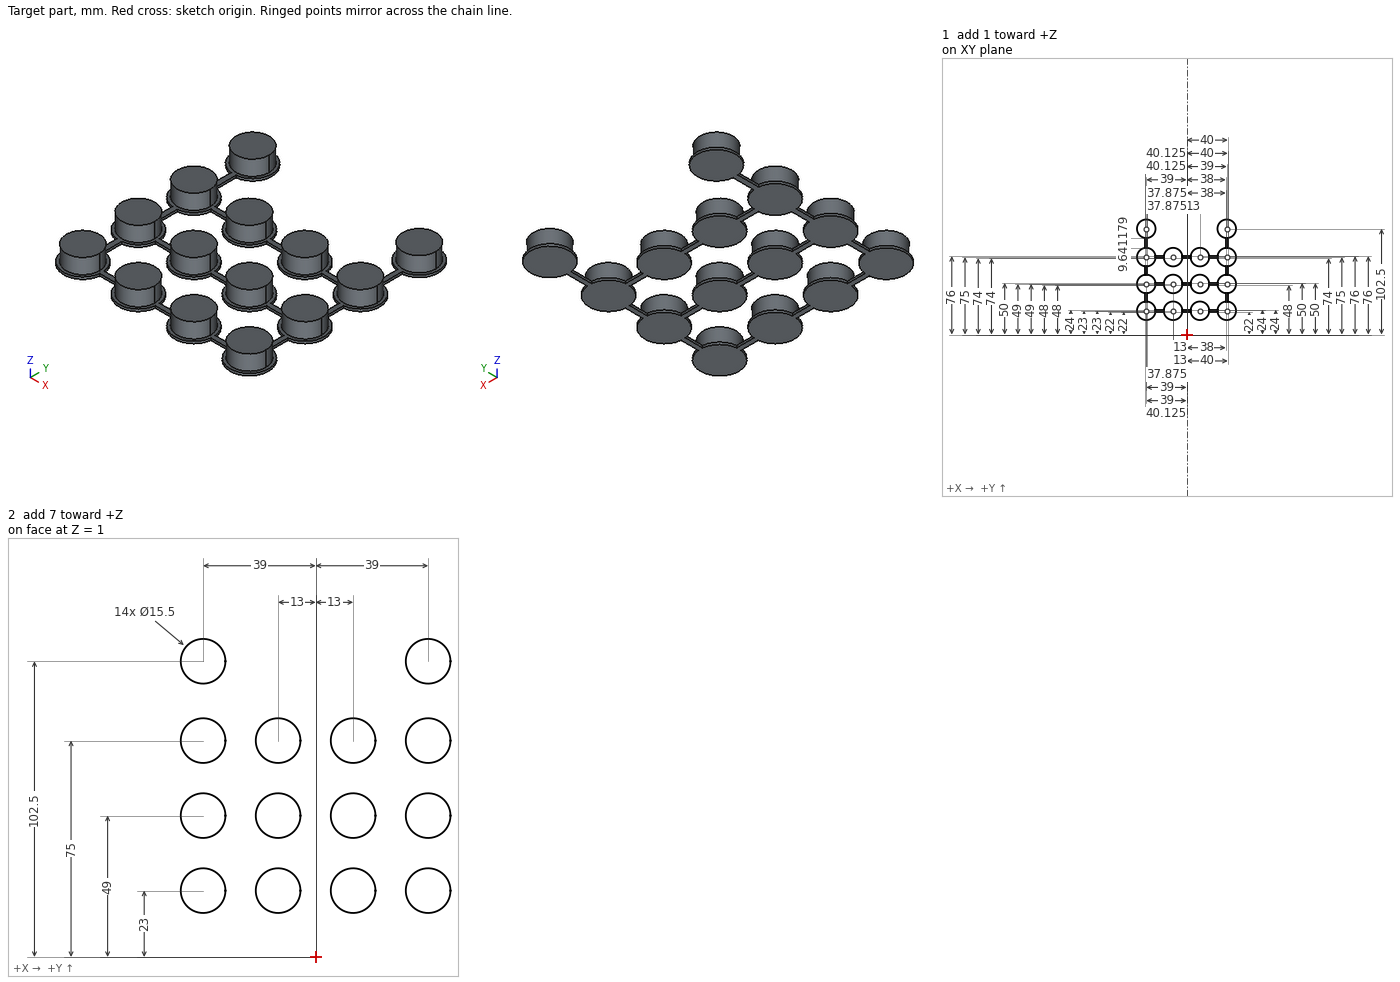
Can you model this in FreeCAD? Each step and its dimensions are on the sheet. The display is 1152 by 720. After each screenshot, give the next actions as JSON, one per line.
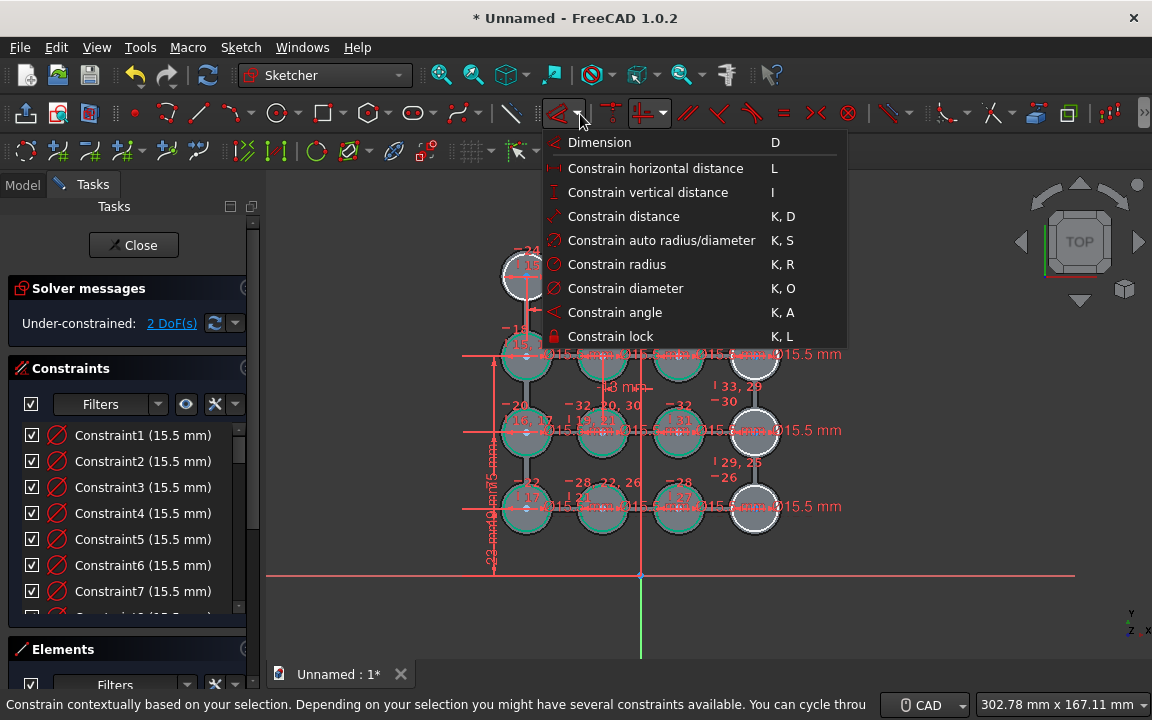
{"action": "left_click", "coordinate": [695, 168]}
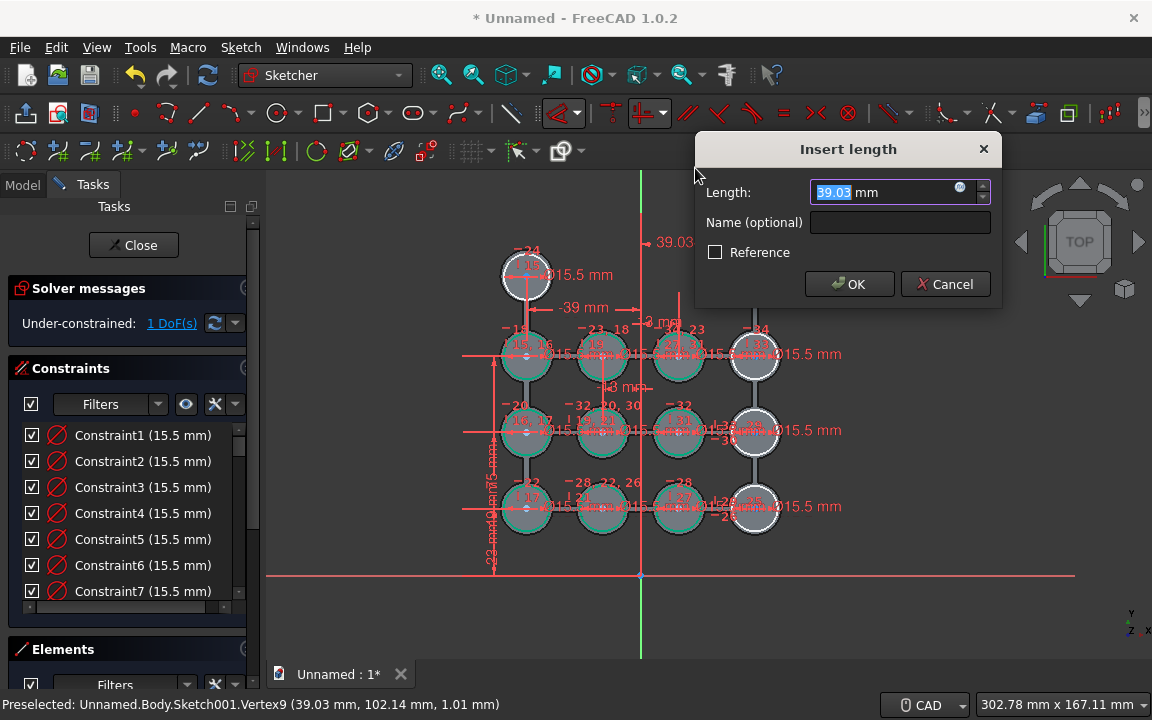
{"action": "type", "text": "39"}
{"action": "key", "text": "Return"}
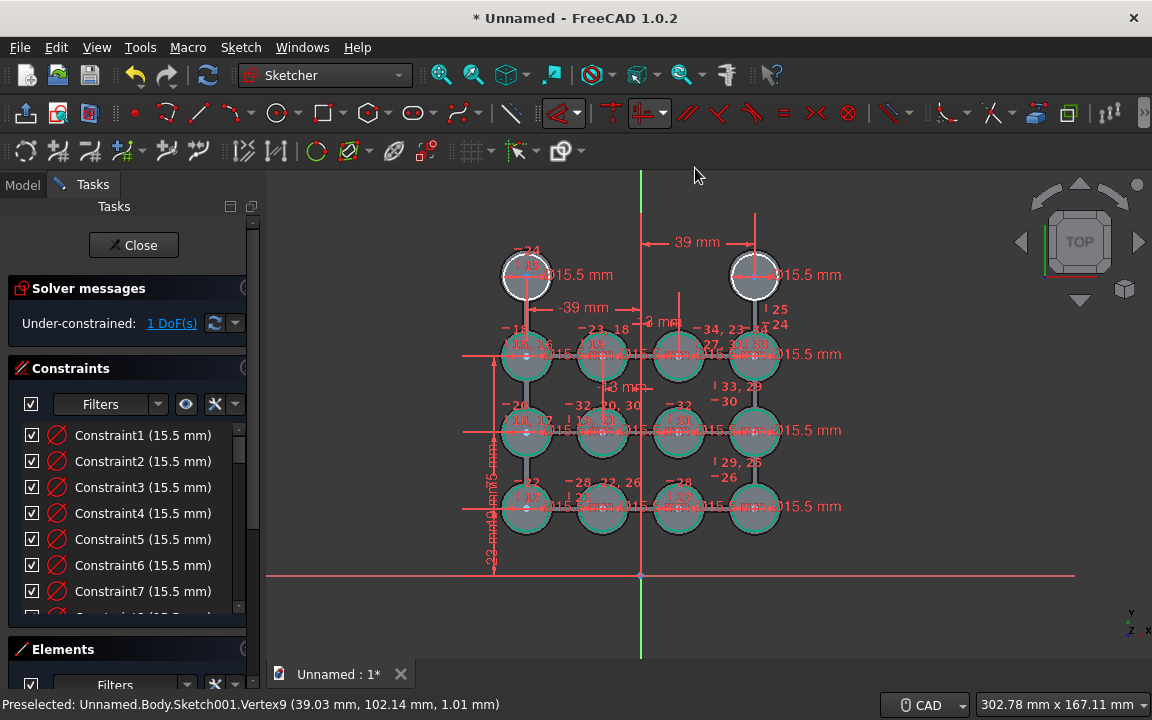
{"action": "left_click", "coordinate": [527, 277]}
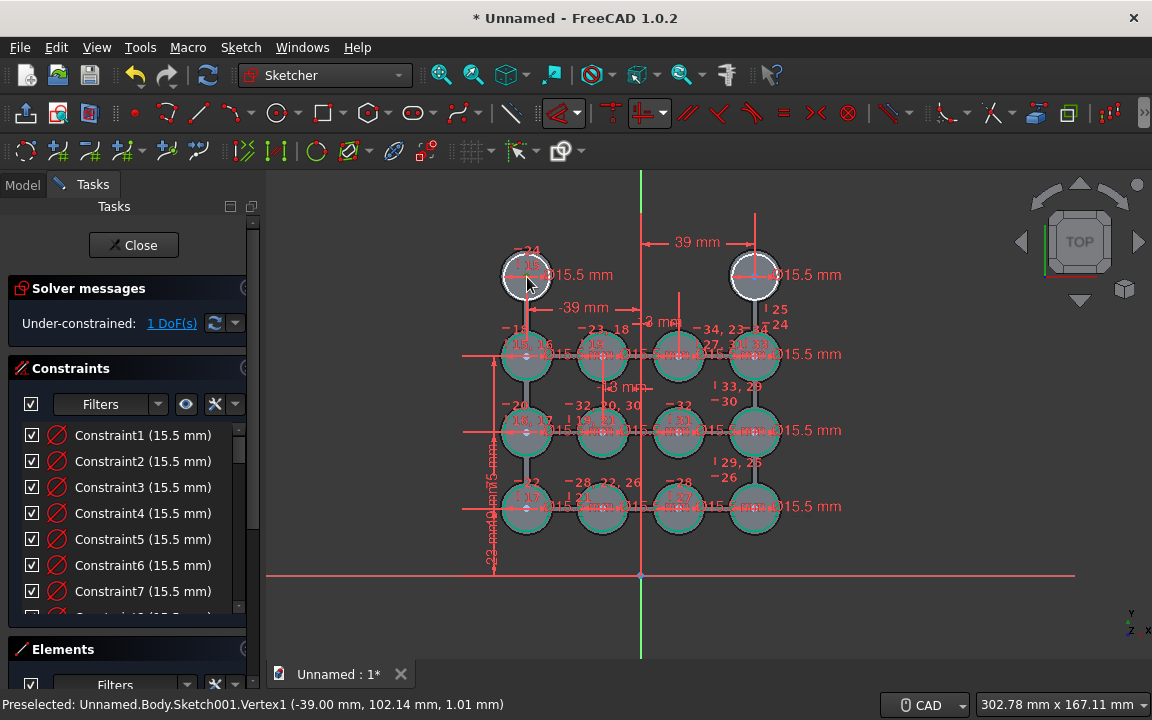
{"action": "left_click", "coordinate": [580, 114]}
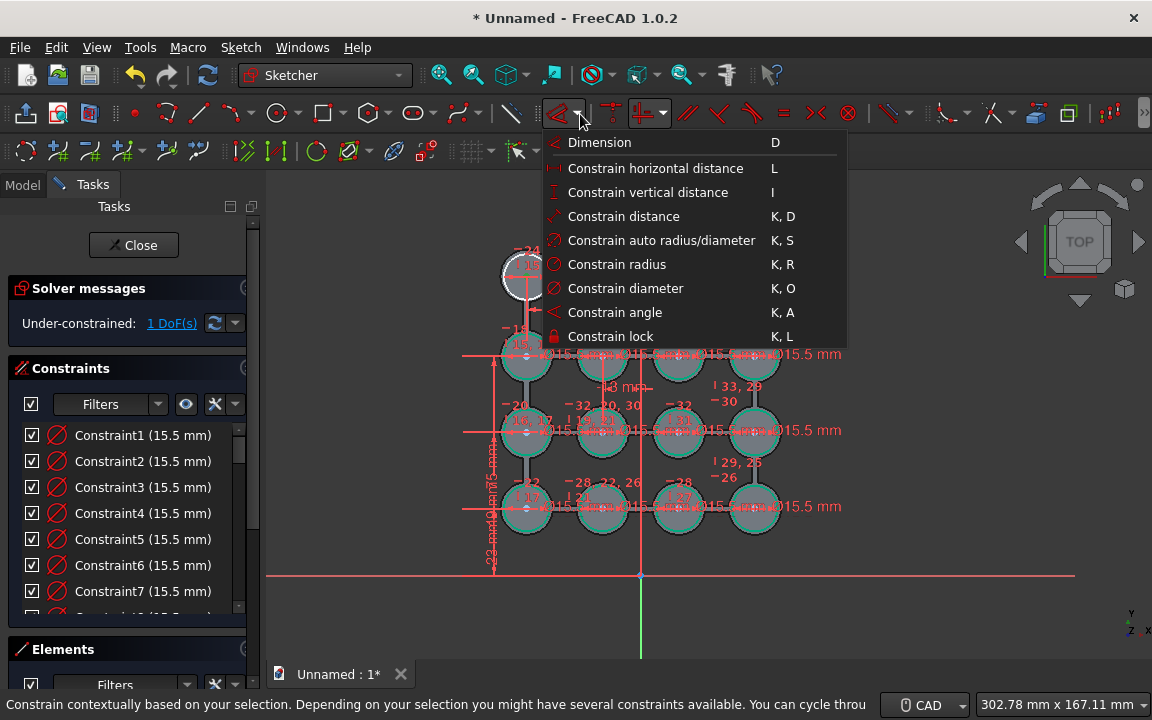
{"action": "left_click", "coordinate": [695, 192]}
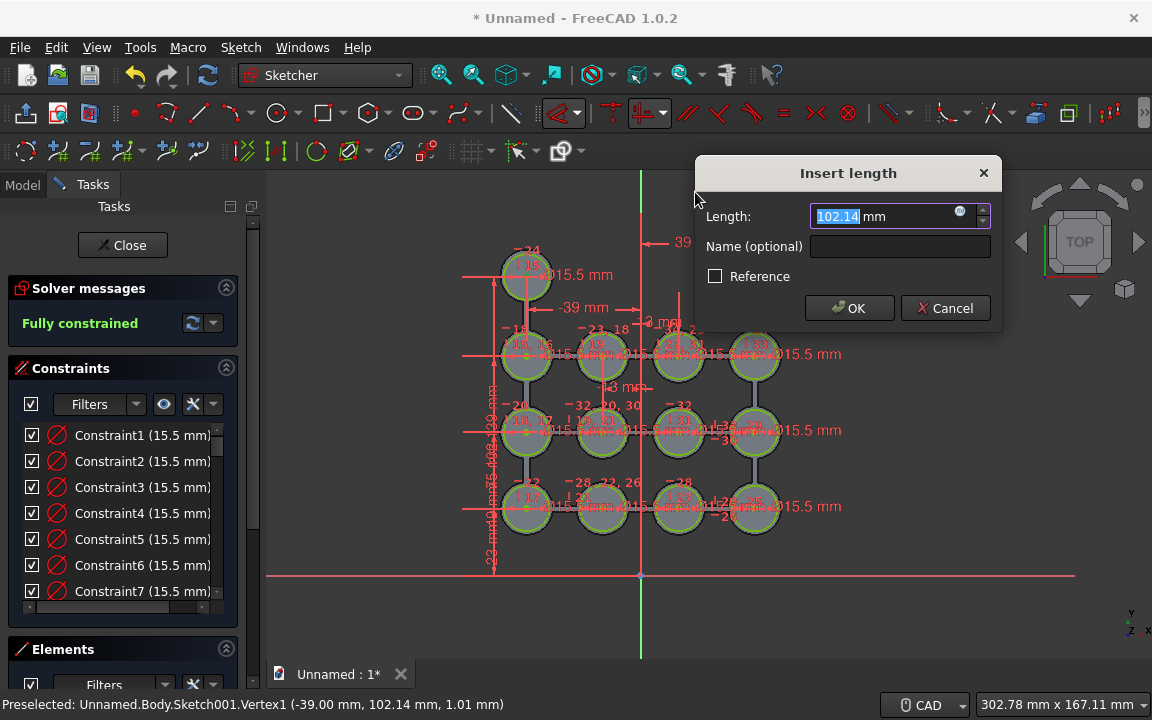
{"action": "type", "text": "102.5"}
{"action": "key", "text": "Return"}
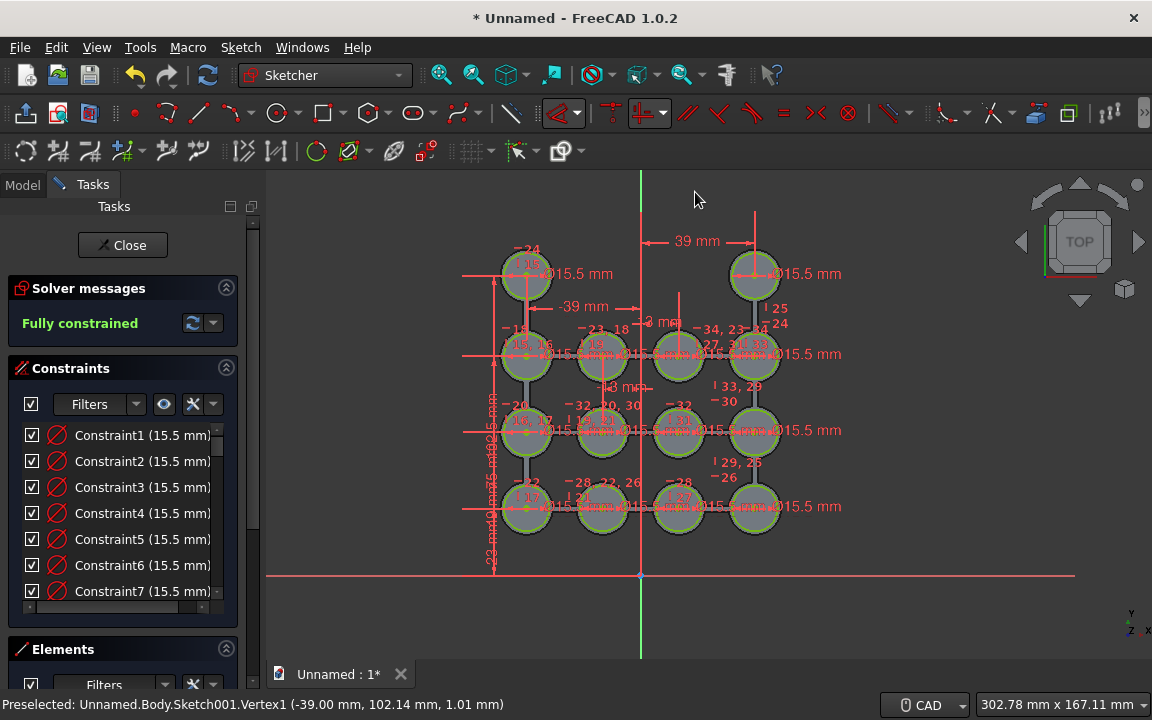
{"action": "left_click", "coordinate": [123, 245]}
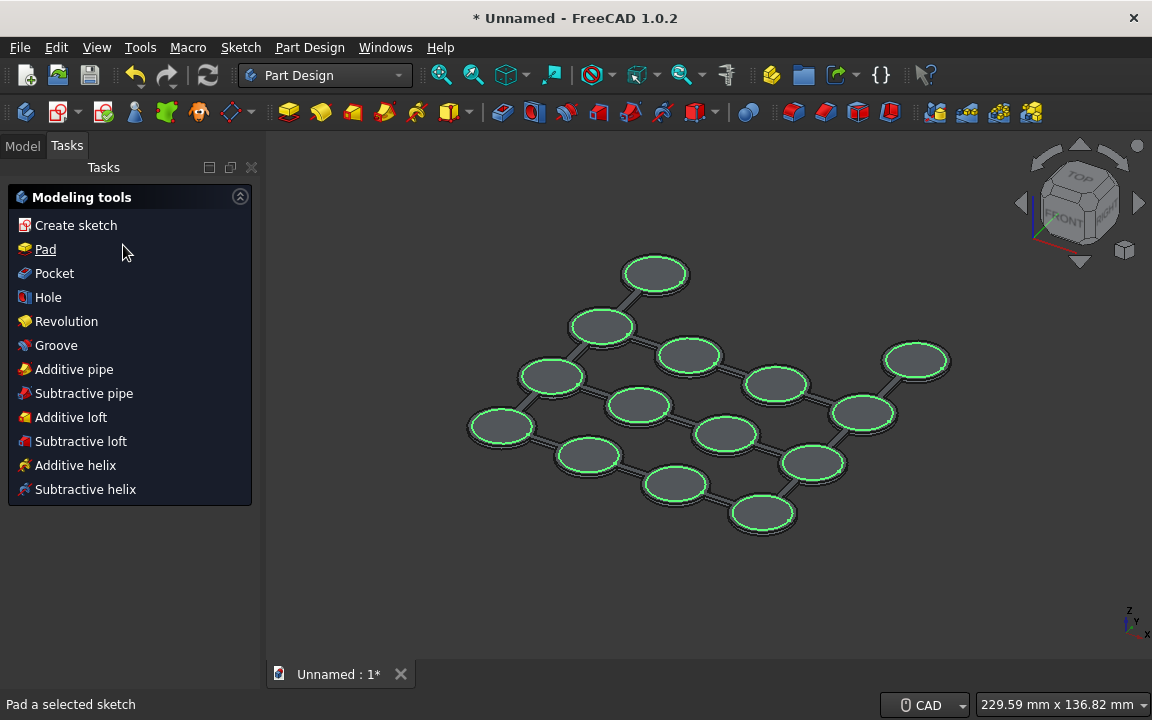
{"action": "left_click", "coordinate": [290, 112]}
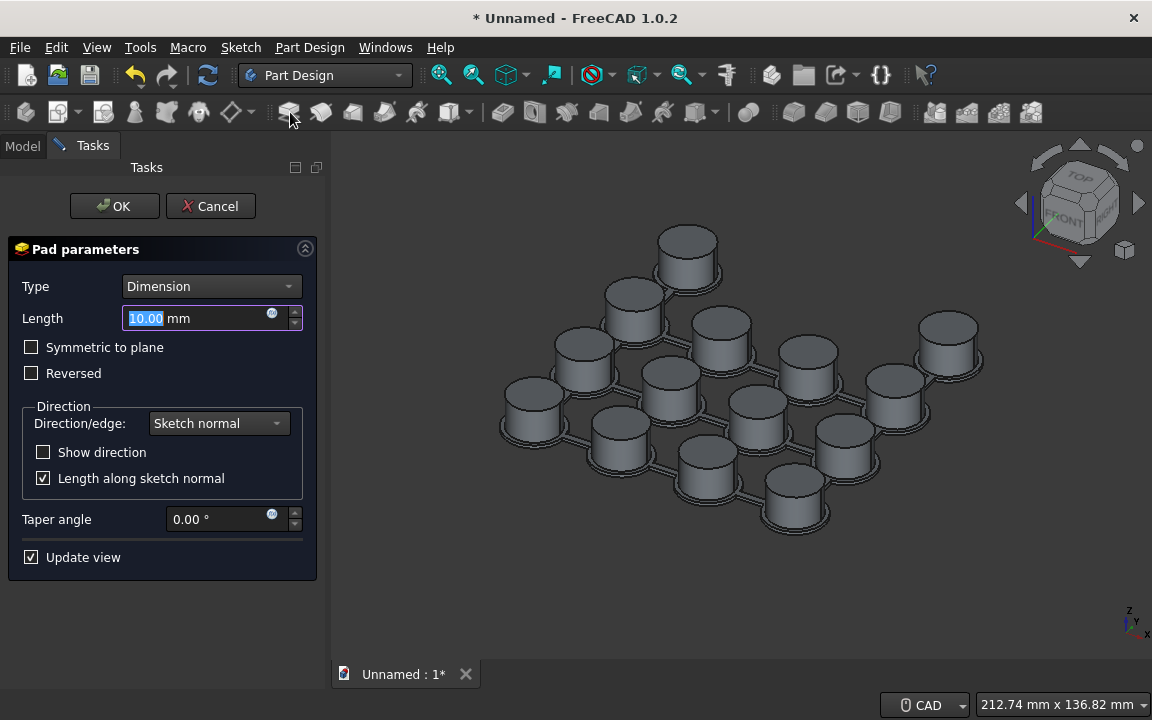
{"action": "type", "text": "7"}
{"action": "key", "text": "Tab"}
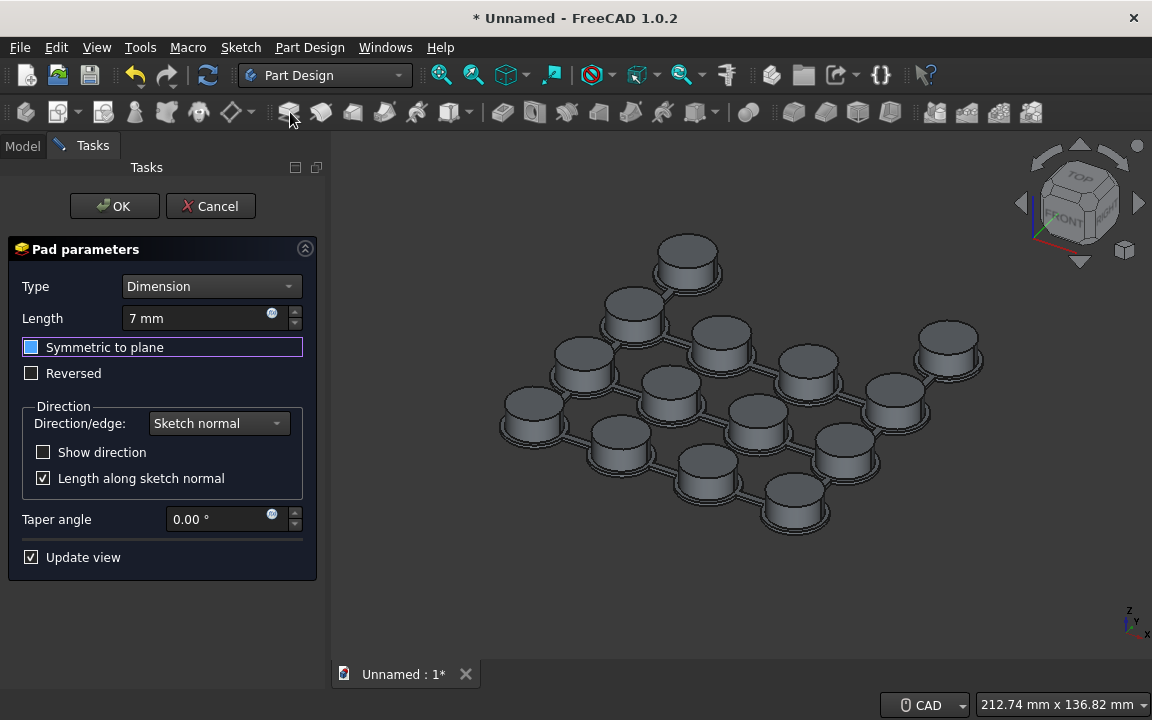
{"action": "left_click", "coordinate": [115, 206]}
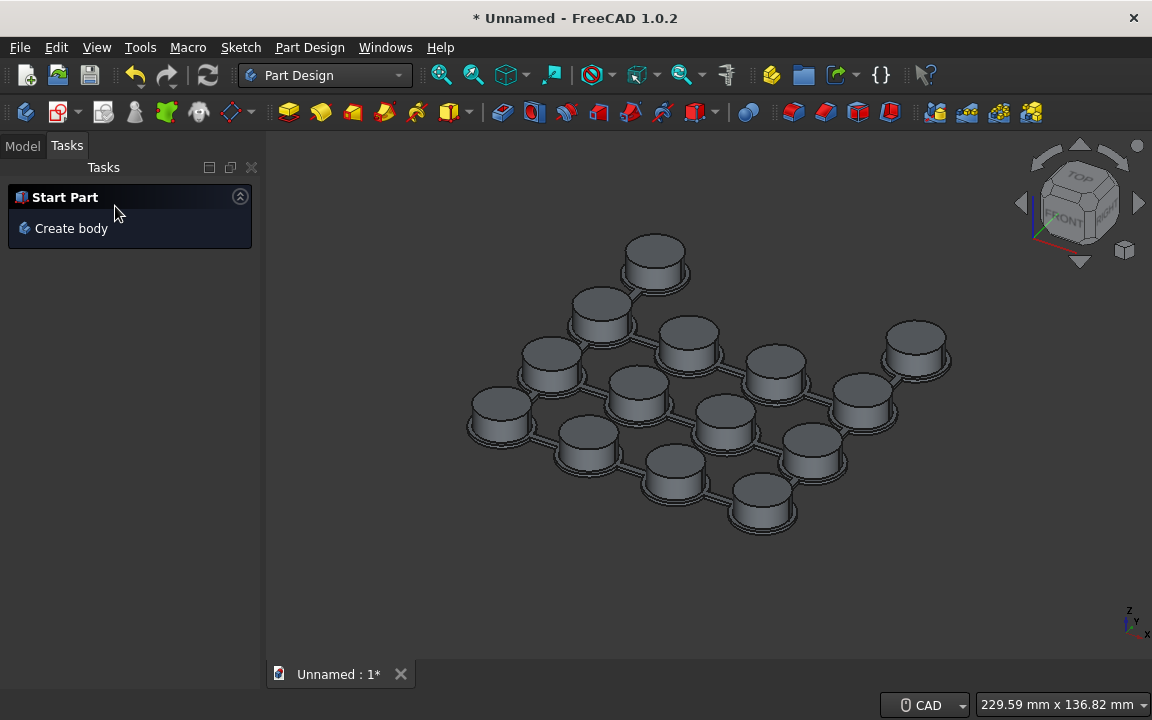
{"action": "key", "text": "0"}